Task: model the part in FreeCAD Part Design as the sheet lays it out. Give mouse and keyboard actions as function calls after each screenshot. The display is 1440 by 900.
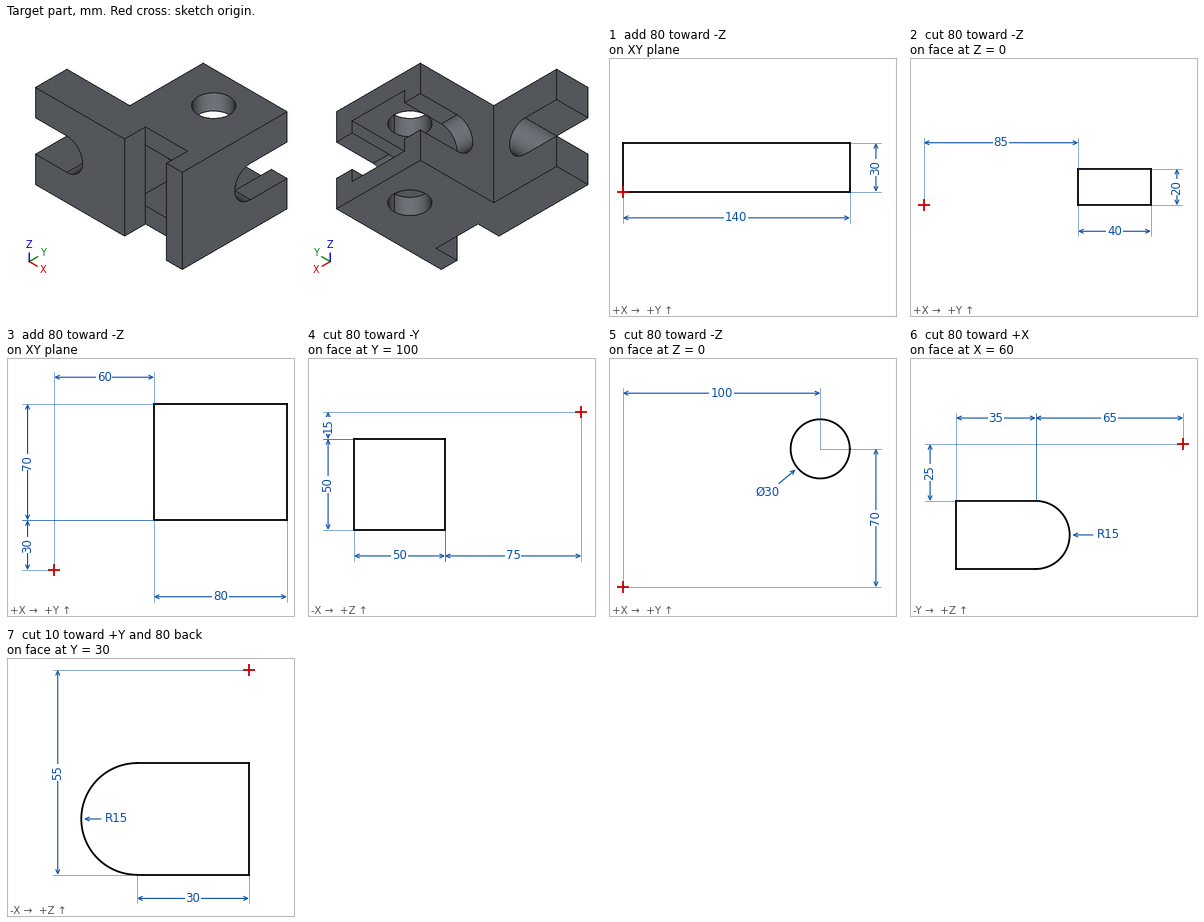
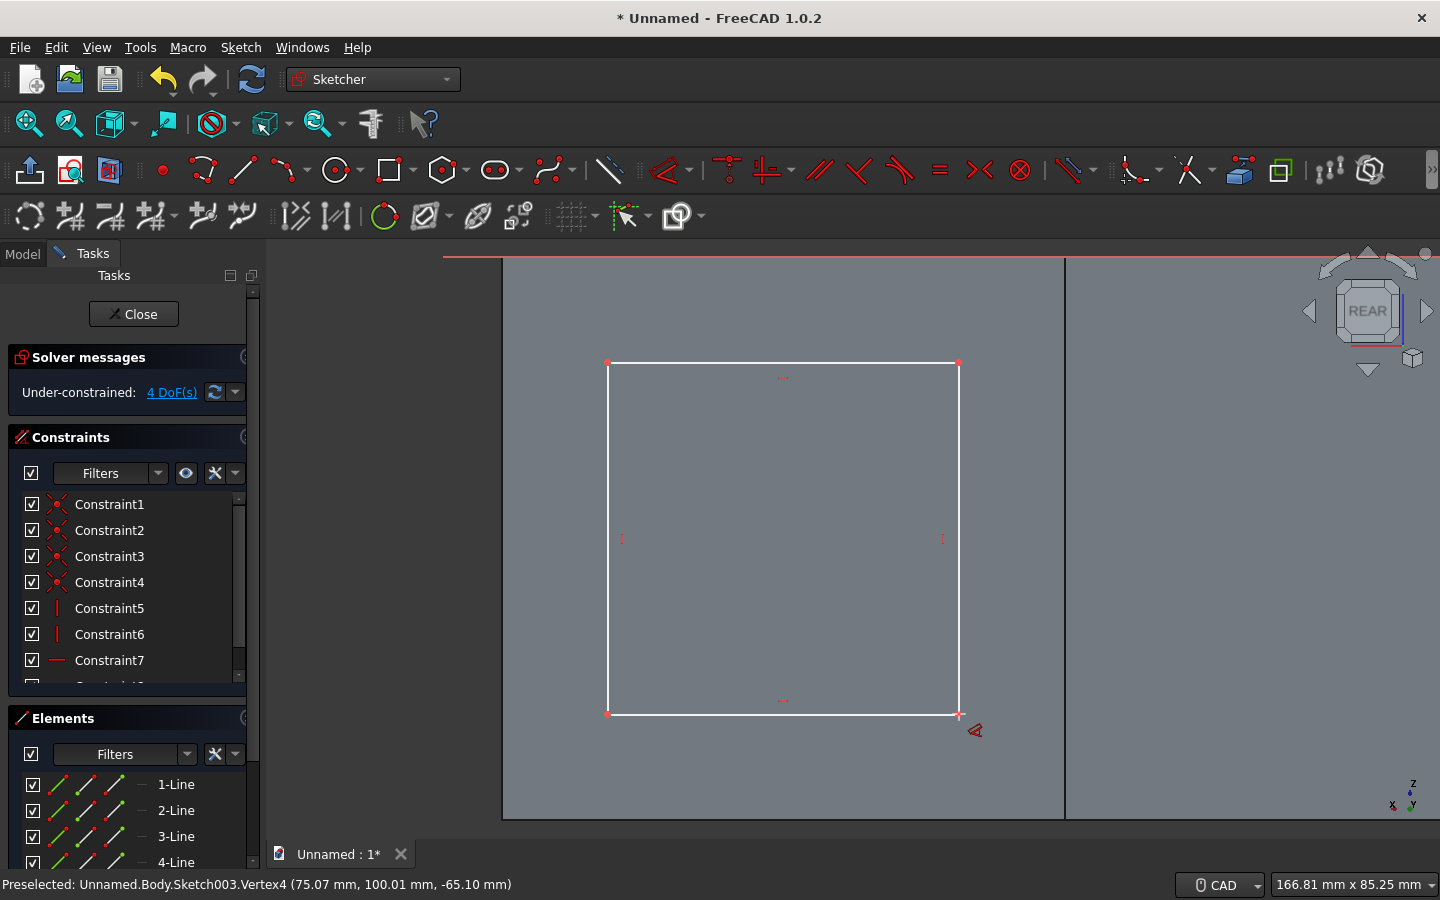
click(608, 469)
click(574, 539)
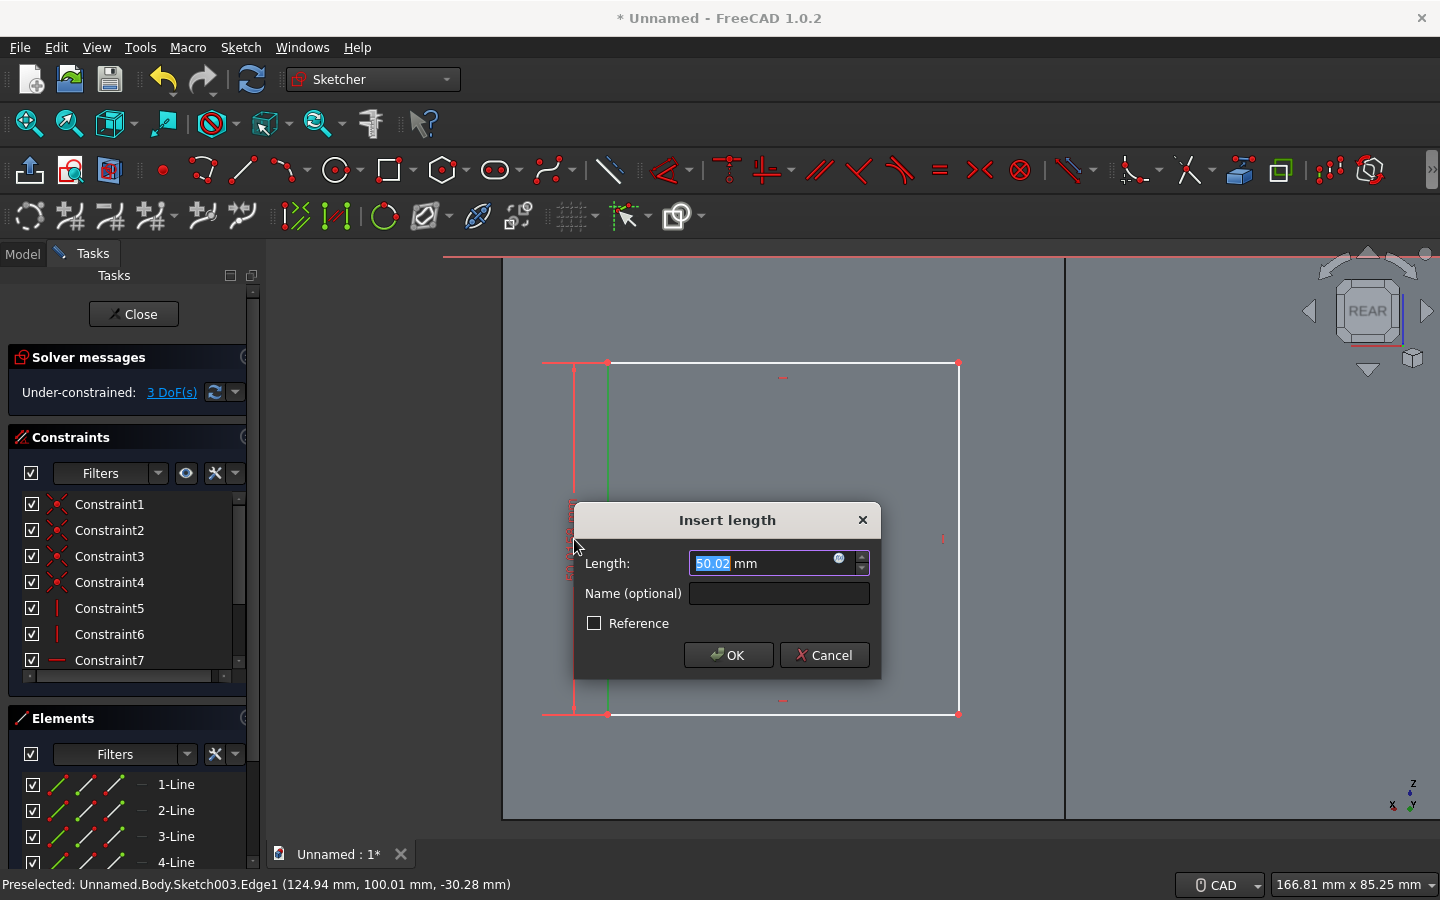
text(50)
key(Return)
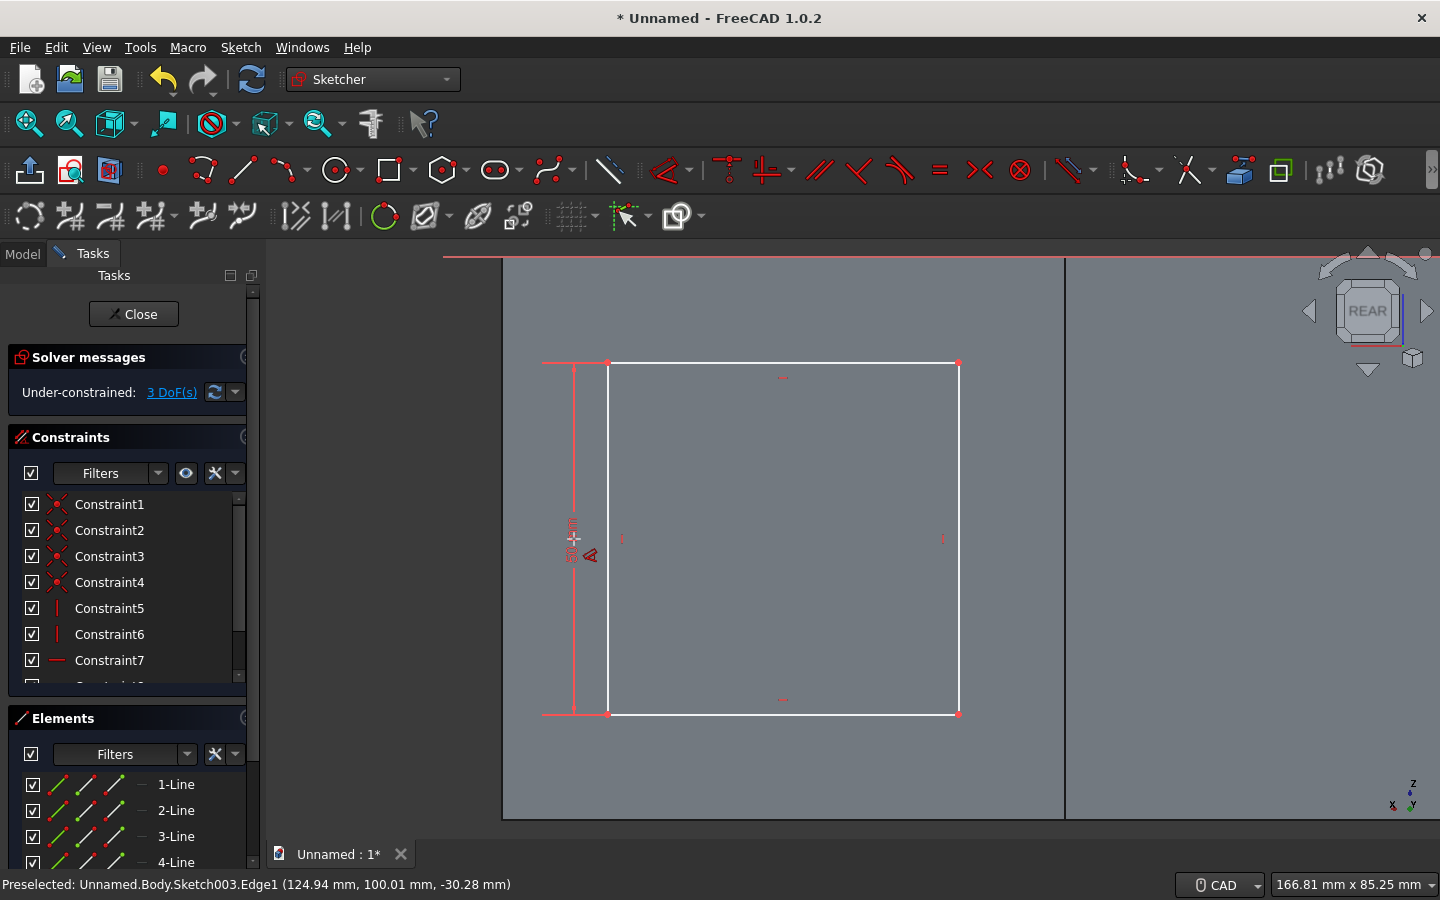
click(713, 715)
click(783, 749)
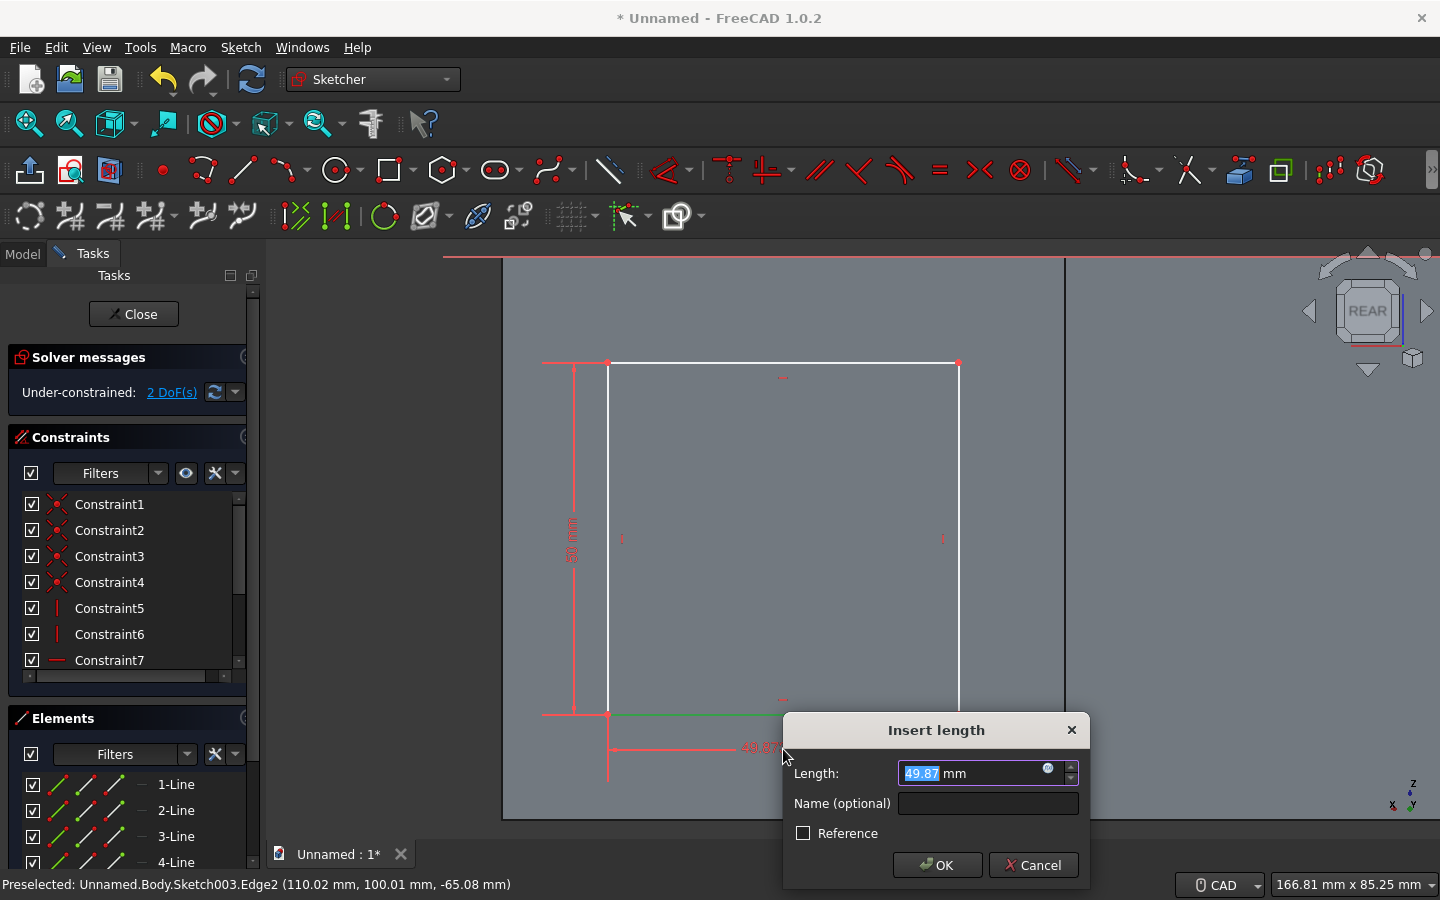
text(50)
key(Return)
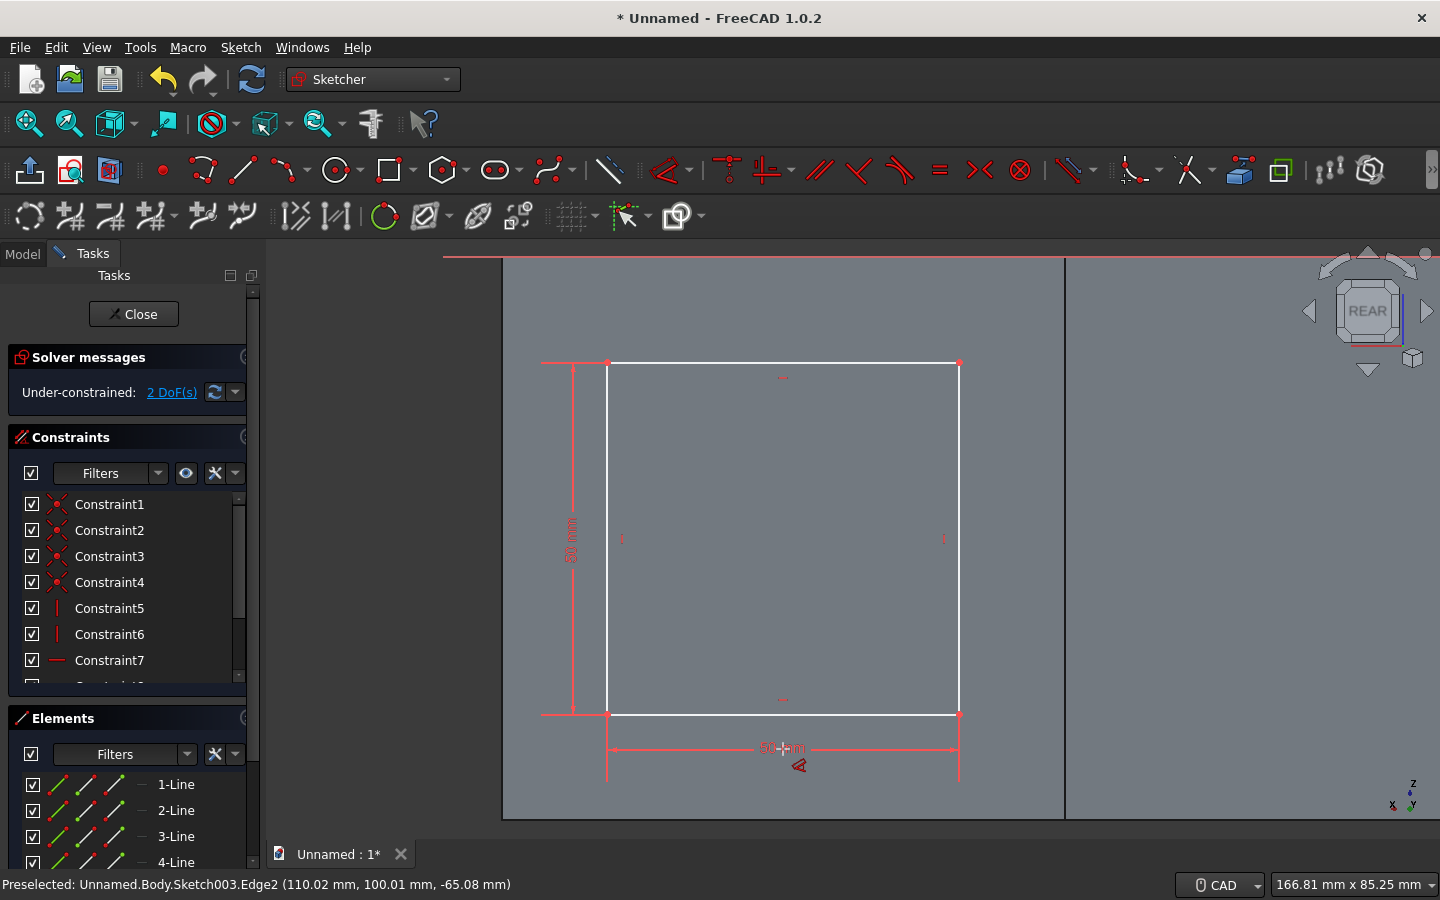
click(607, 363)
click(573, 315)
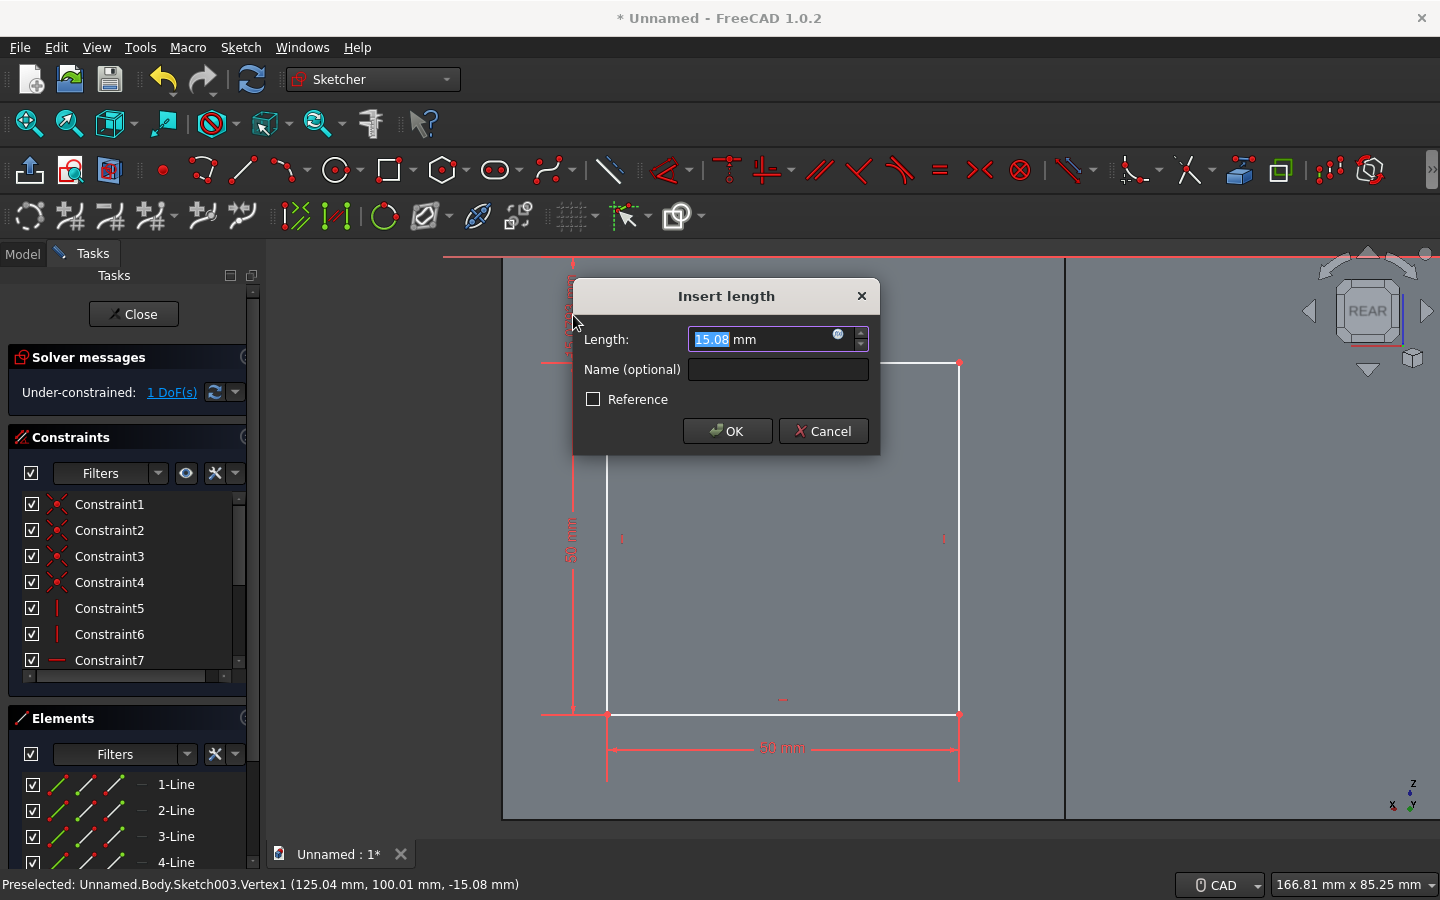
text(15)
key(Return)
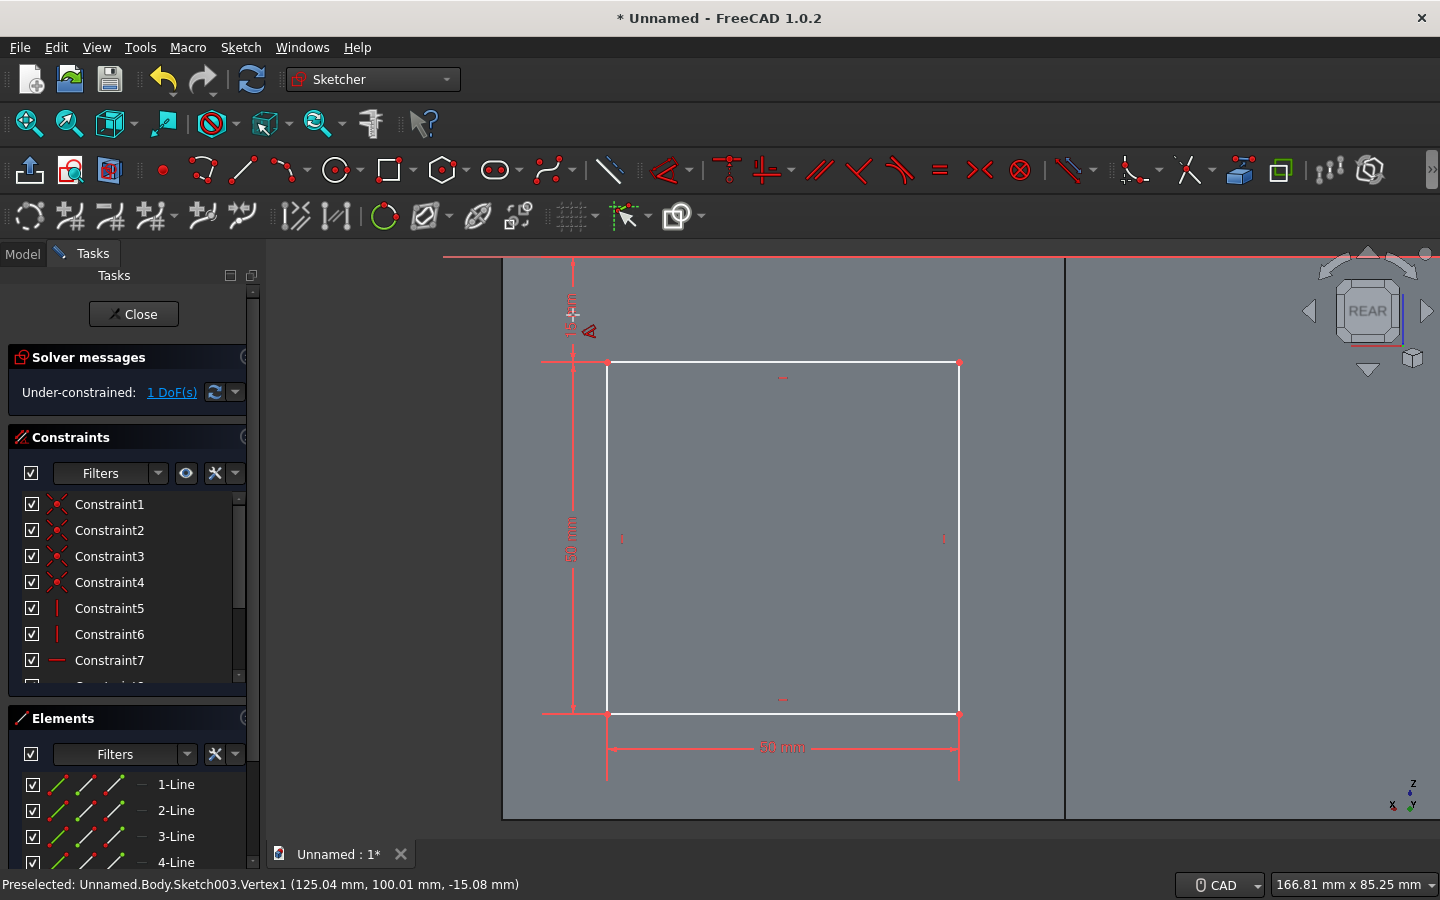
click(959, 714)
click(1117, 748)